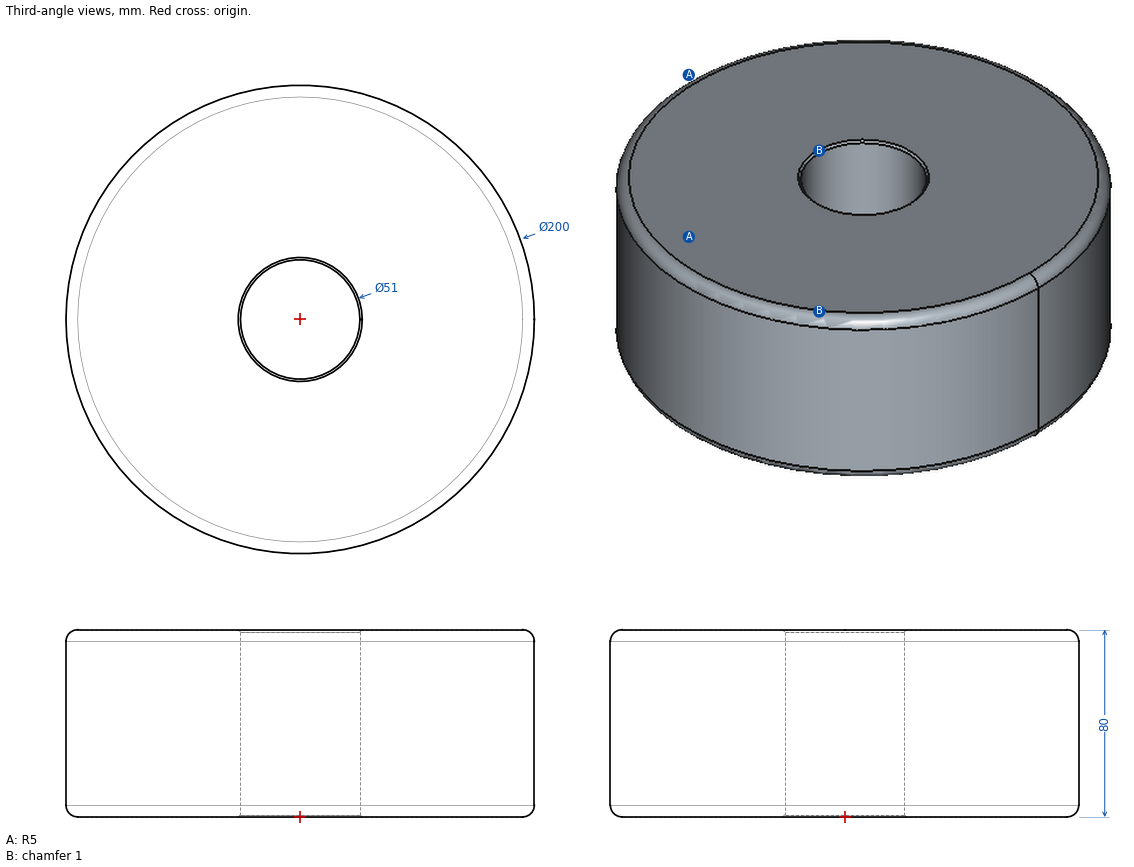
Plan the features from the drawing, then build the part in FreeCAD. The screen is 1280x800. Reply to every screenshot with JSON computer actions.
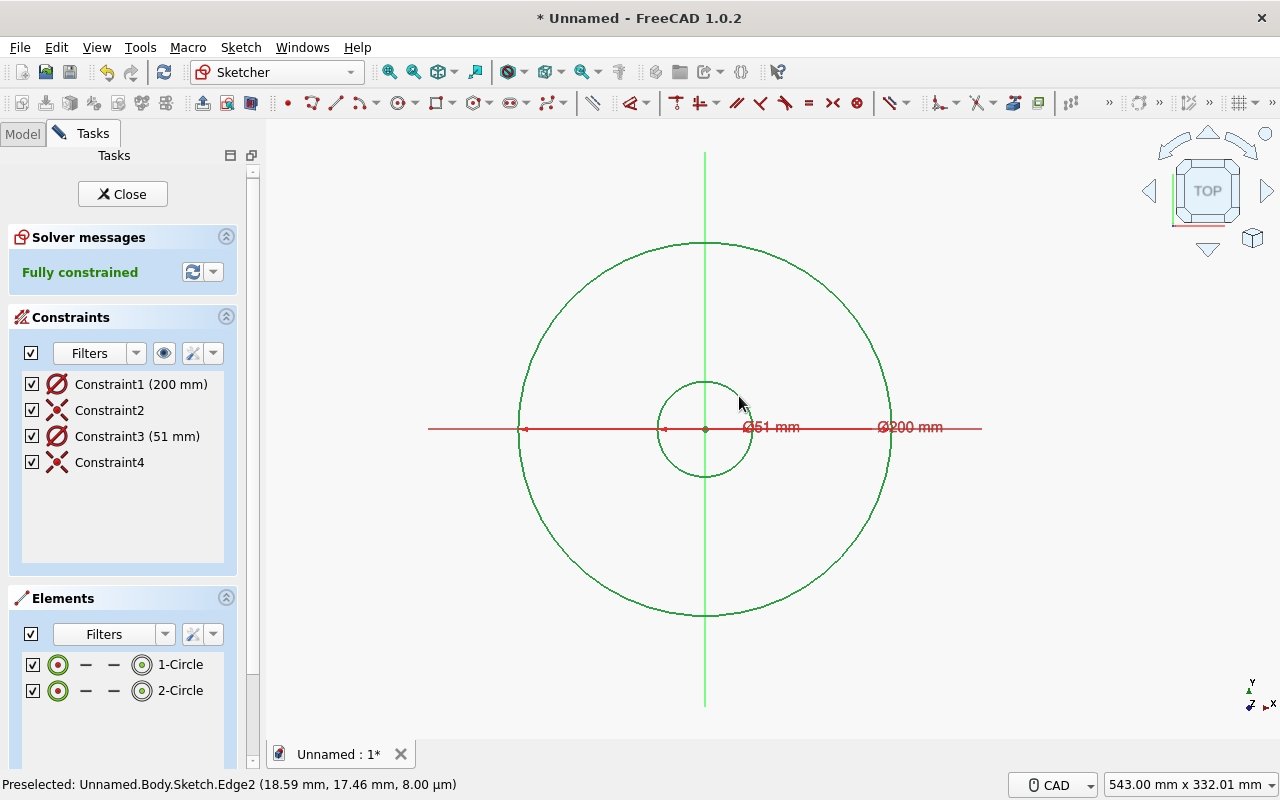
{"action": "left_click", "coordinate": [123, 194]}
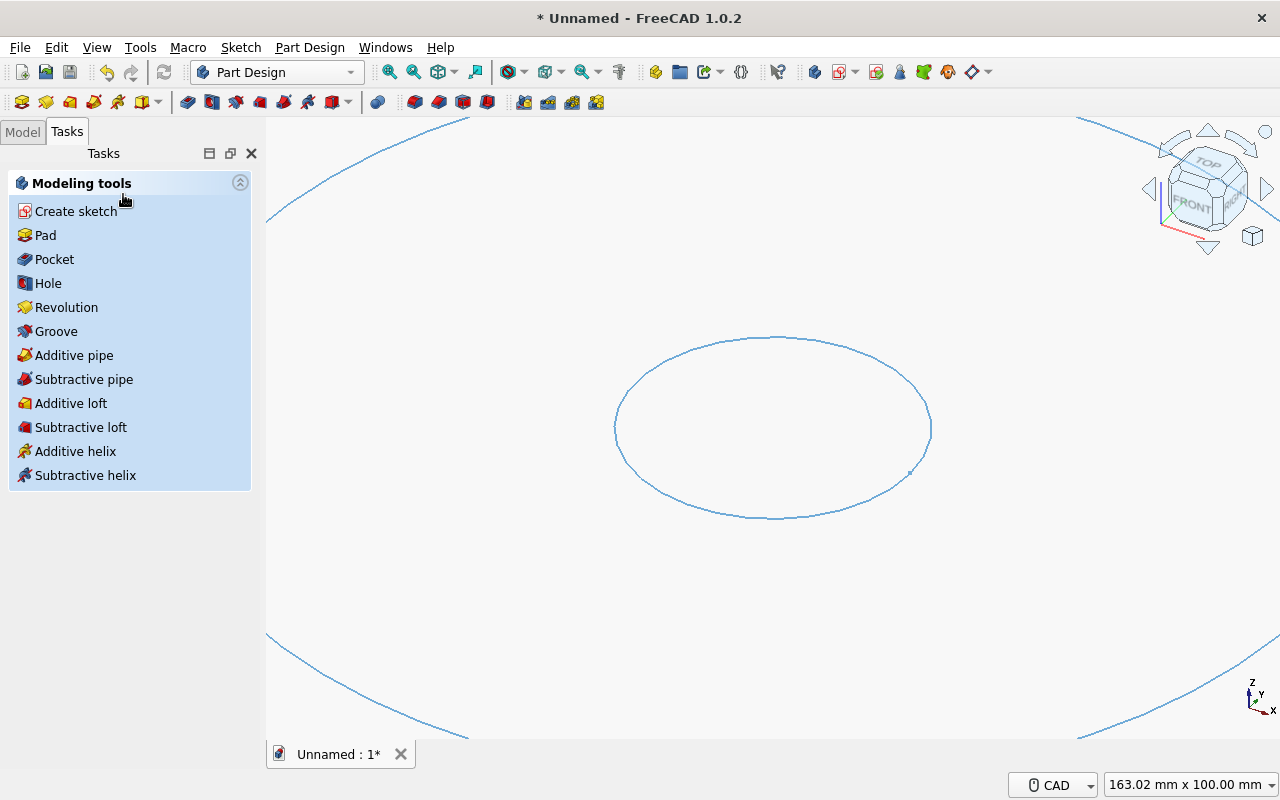
{"action": "left_click", "coordinate": [22, 102]}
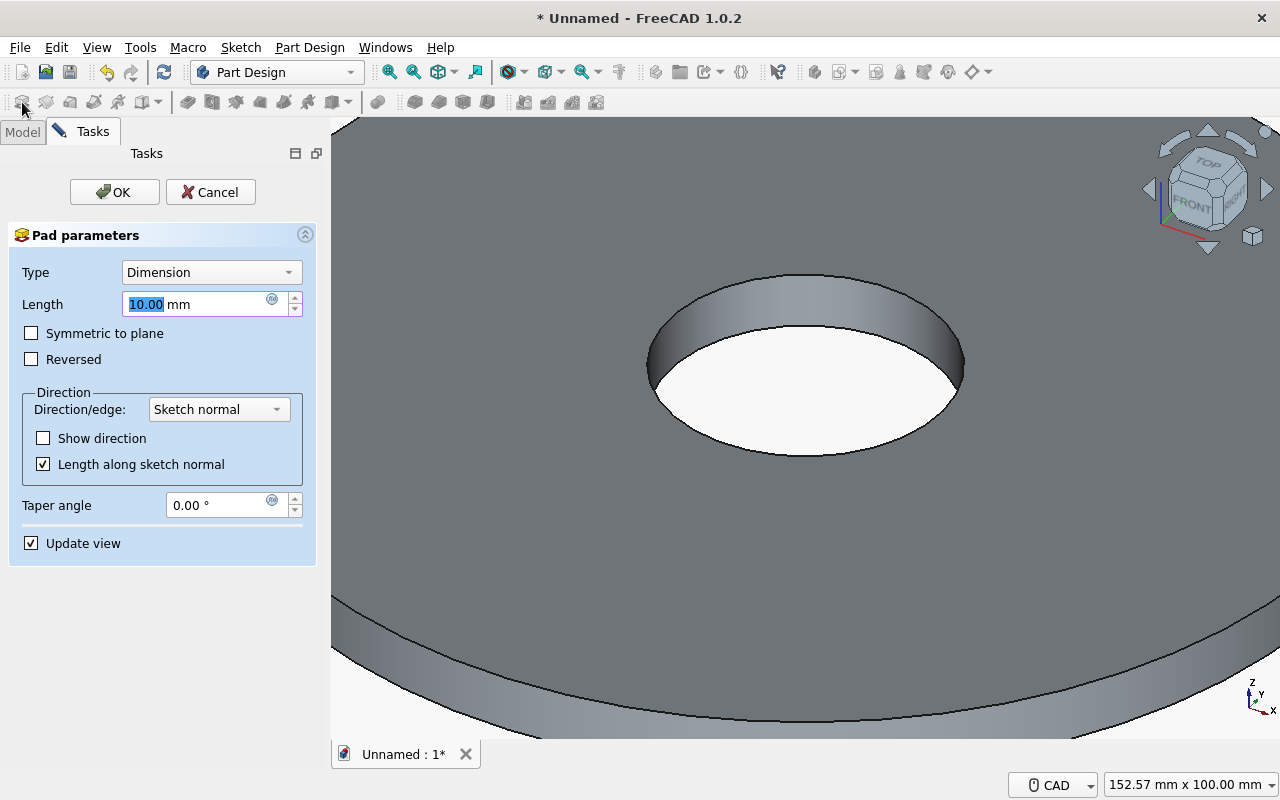
{"action": "type", "text": "80"}
{"action": "key", "text": "Tab"}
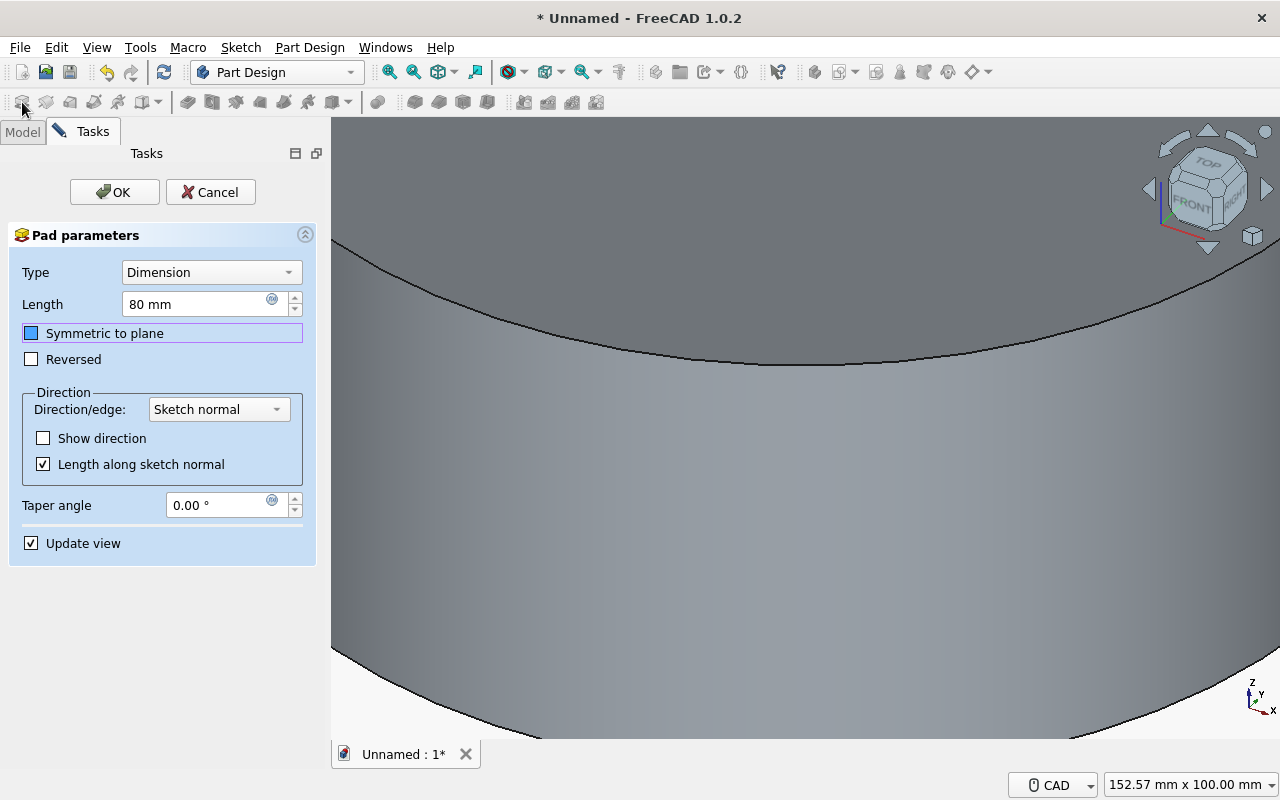
{"action": "left_click", "coordinate": [115, 192]}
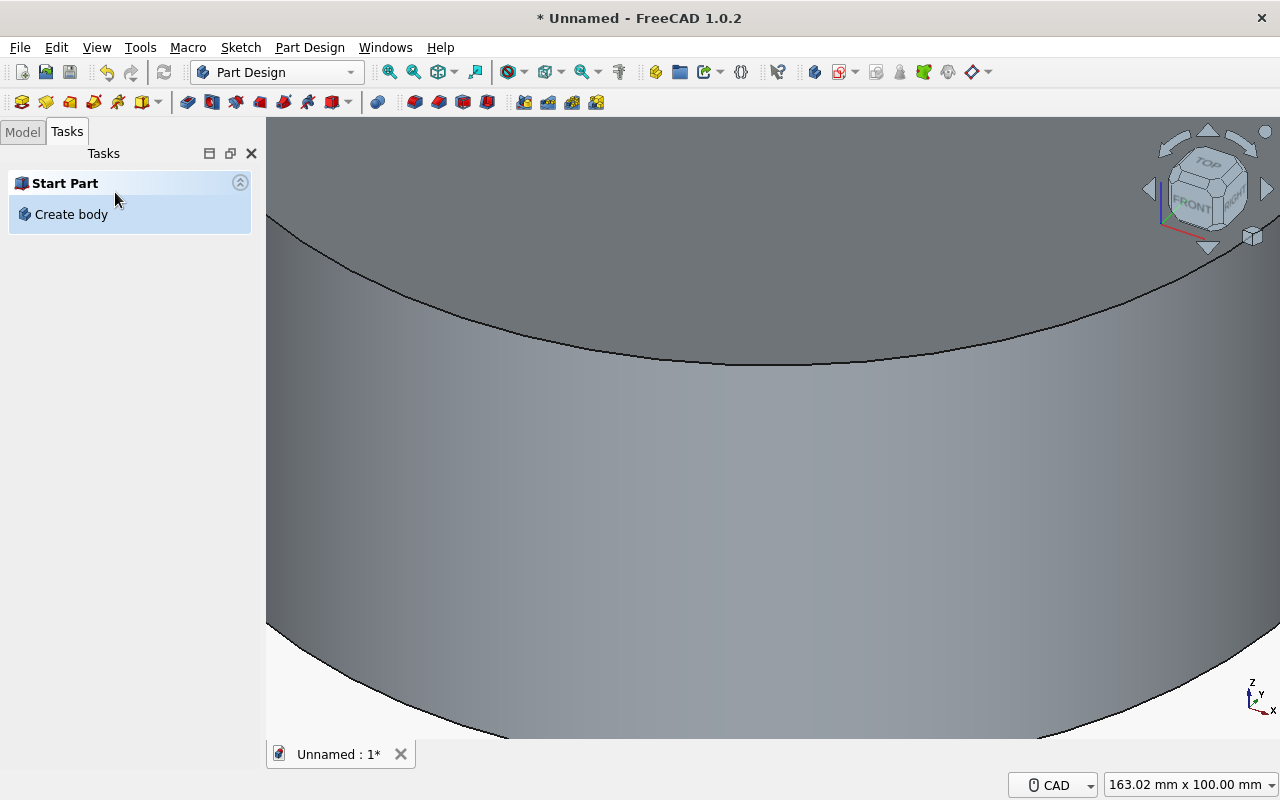
{"action": "left_click", "coordinate": [390, 72]}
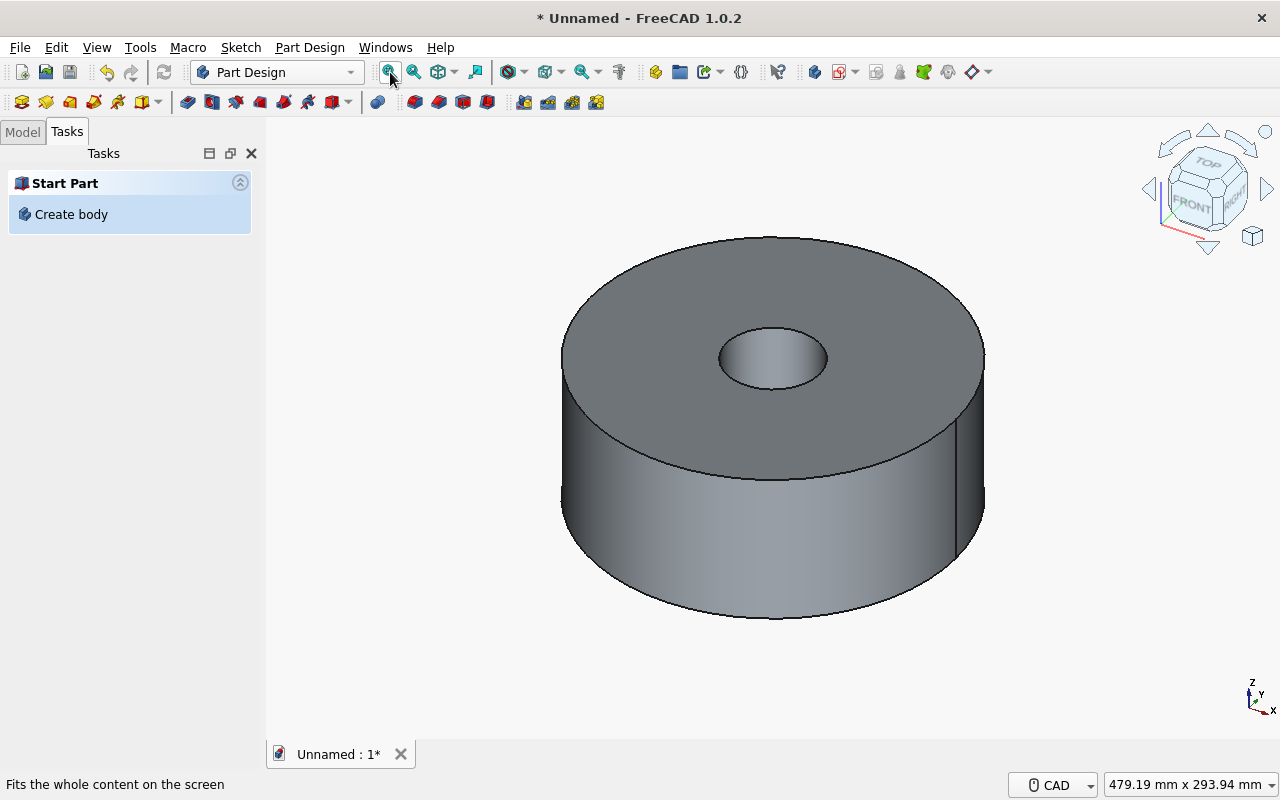
{"action": "left_click", "coordinate": [563, 370]}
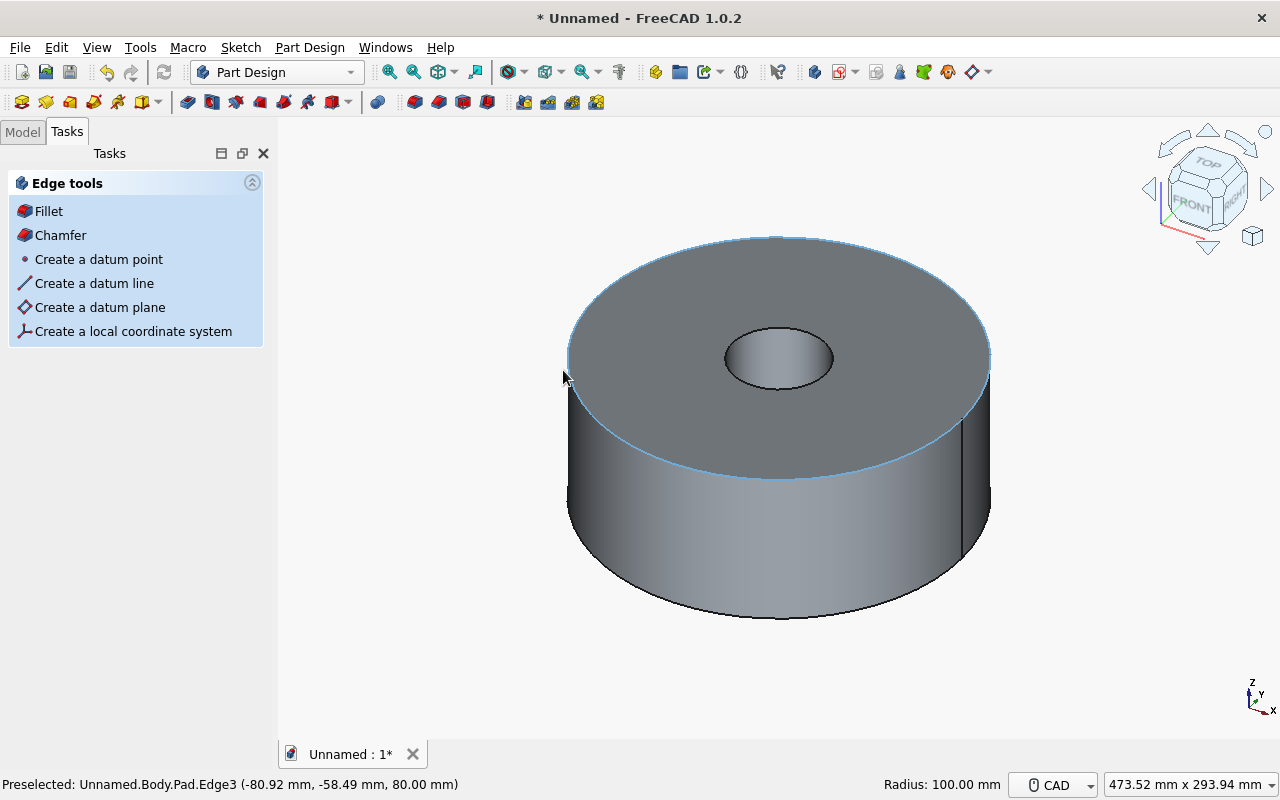
{"action": "key", "text": "0"}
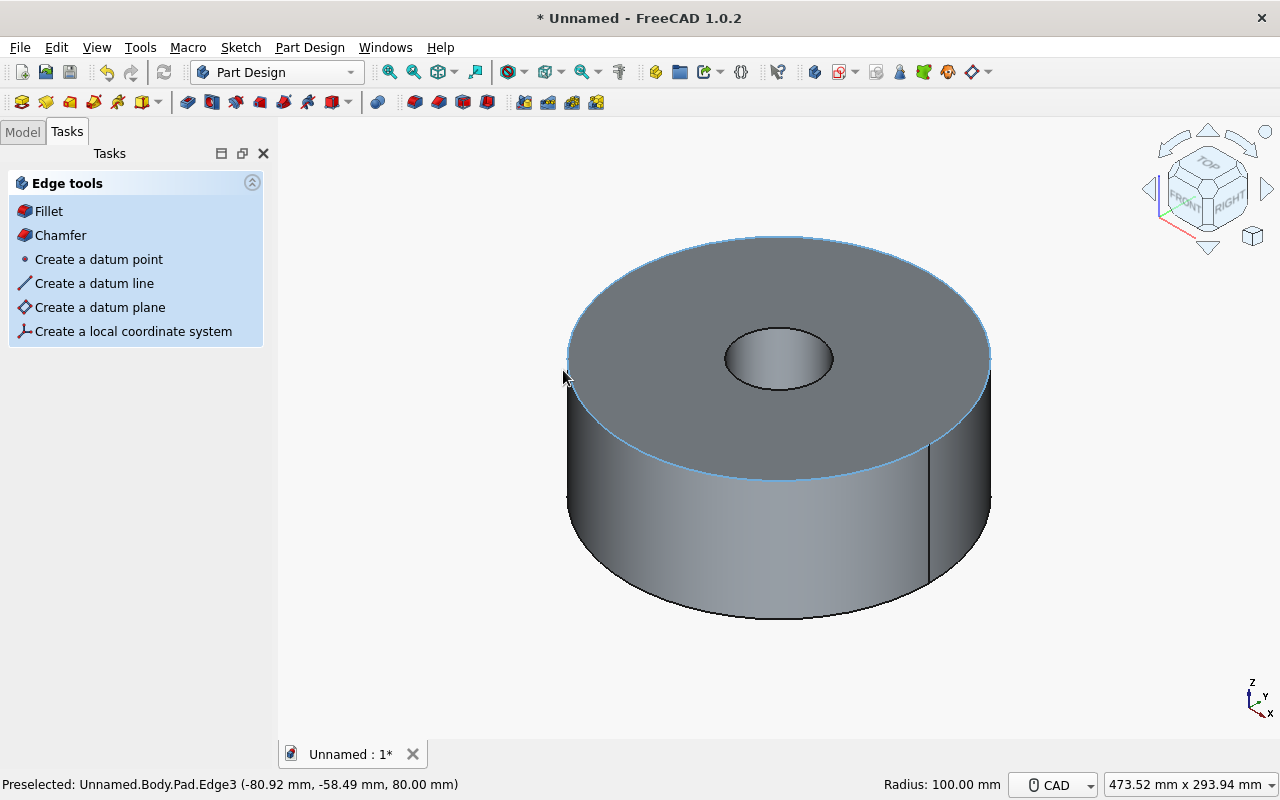
{"action": "key", "text": "2"}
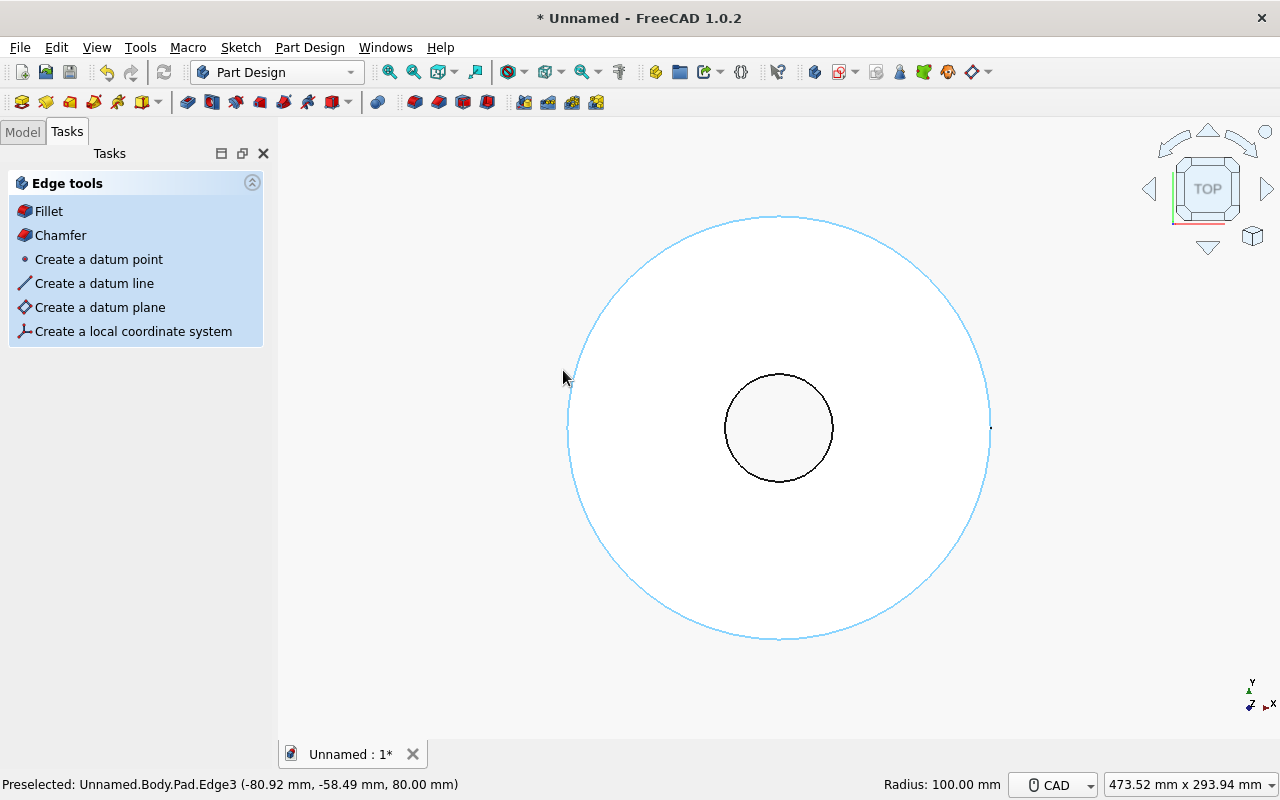
{"action": "key", "text": "1"}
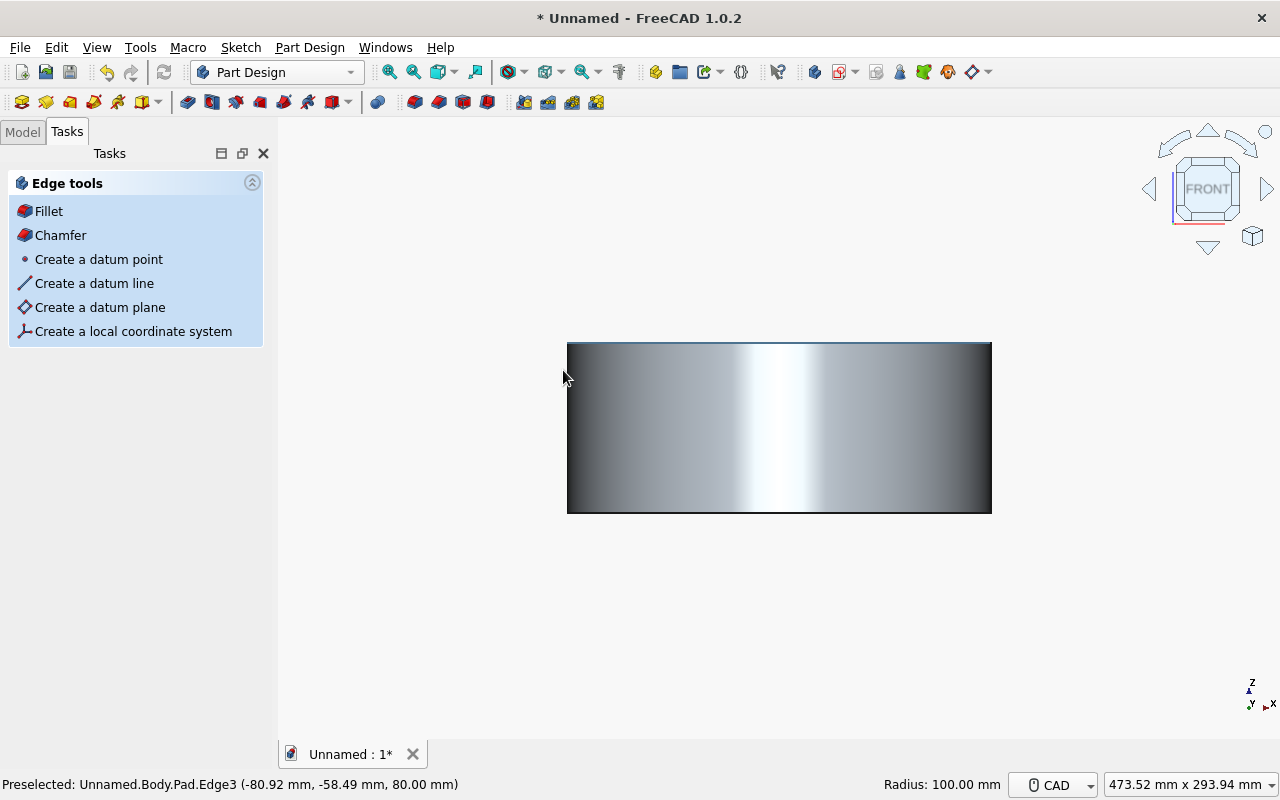
{"action": "left_click", "coordinate": [390, 72]}